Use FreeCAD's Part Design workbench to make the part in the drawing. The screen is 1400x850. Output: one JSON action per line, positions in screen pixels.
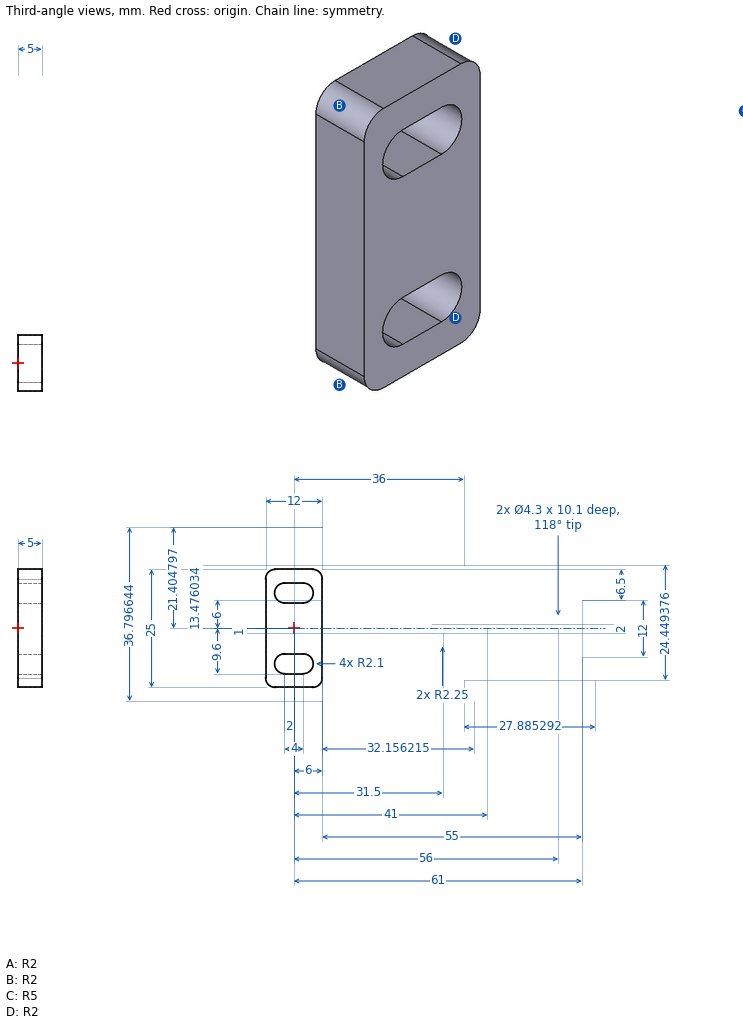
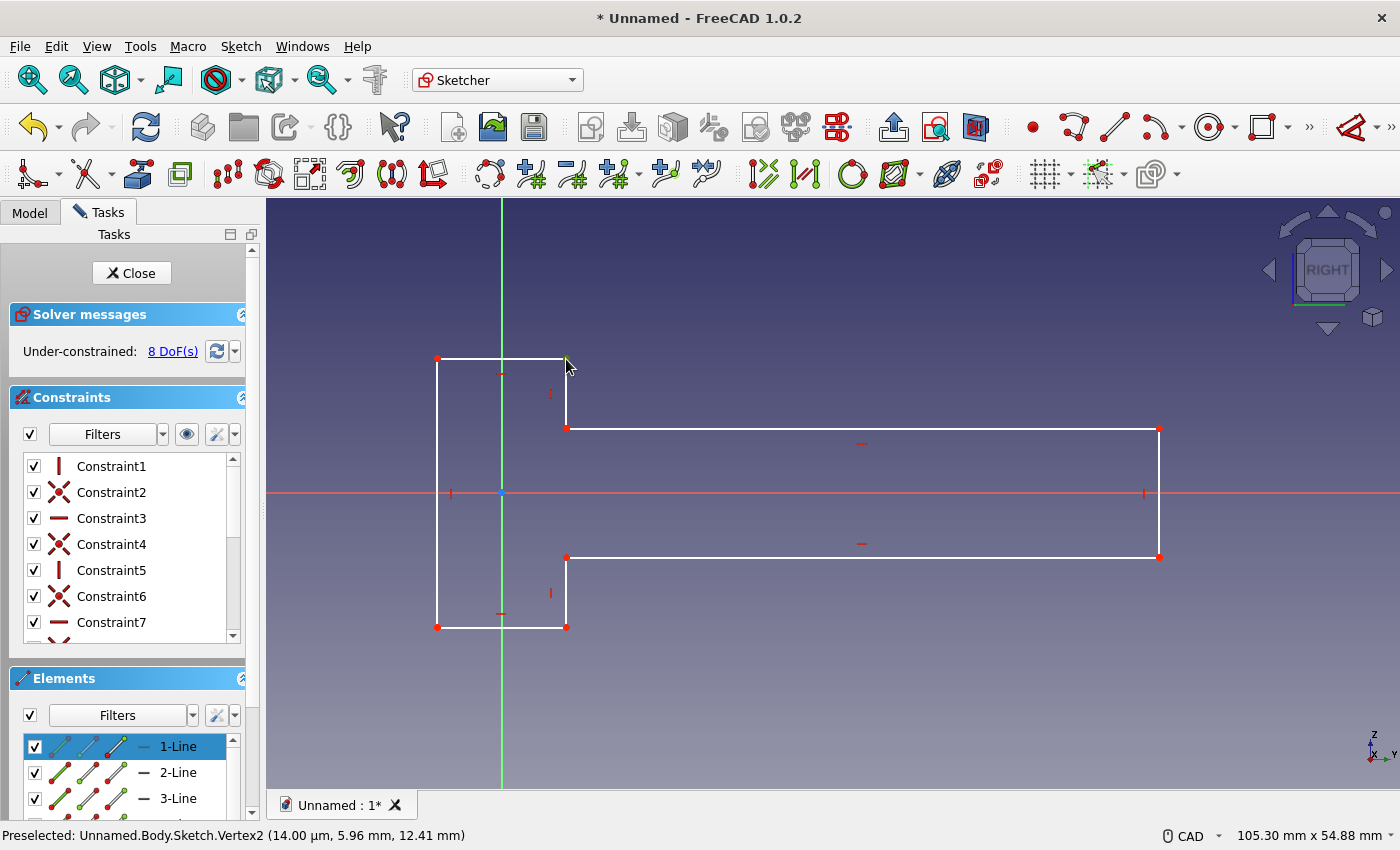
{"action": "left_click", "coordinate": [566, 628]}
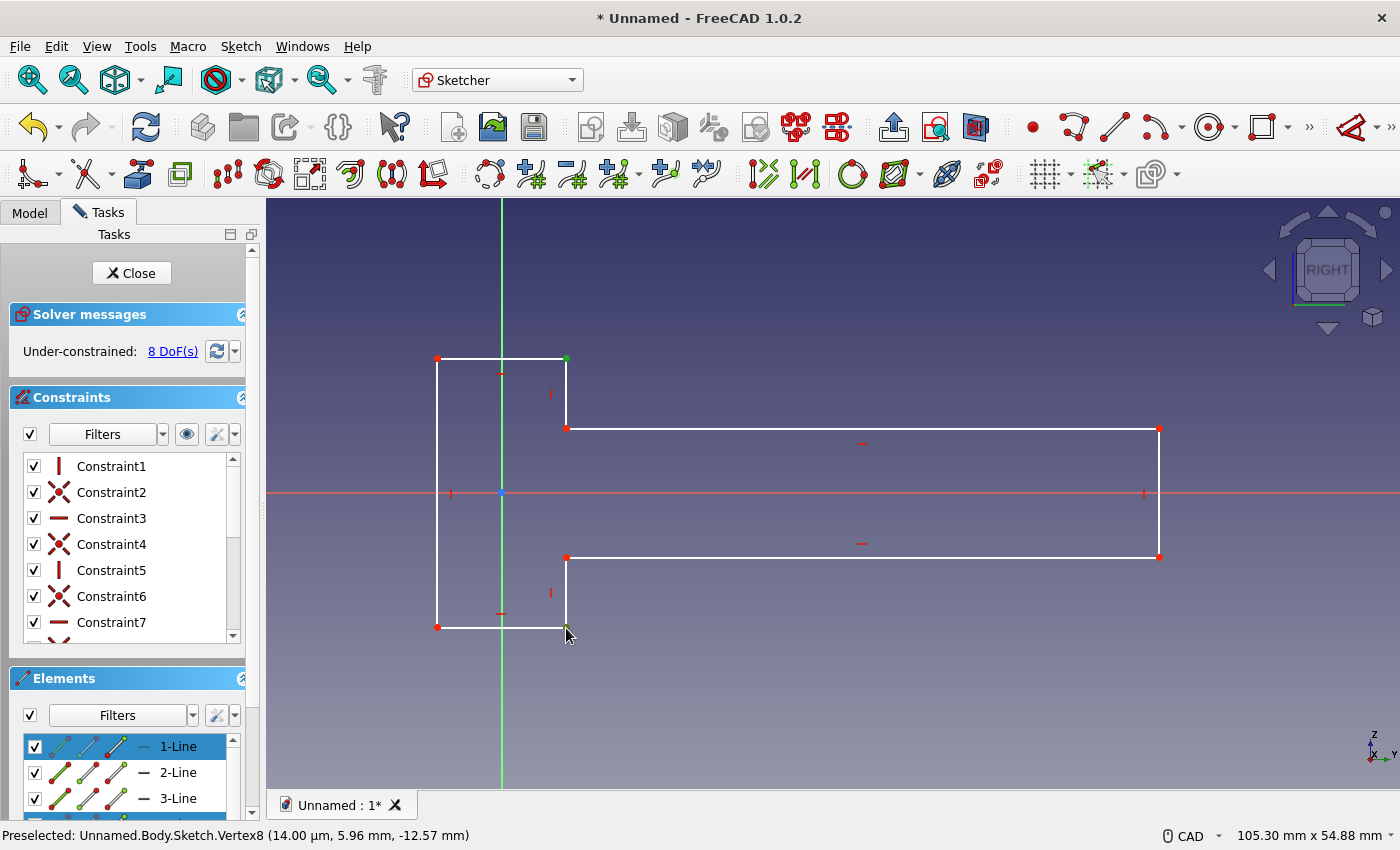
{"action": "left_click", "coordinate": [361, 493]}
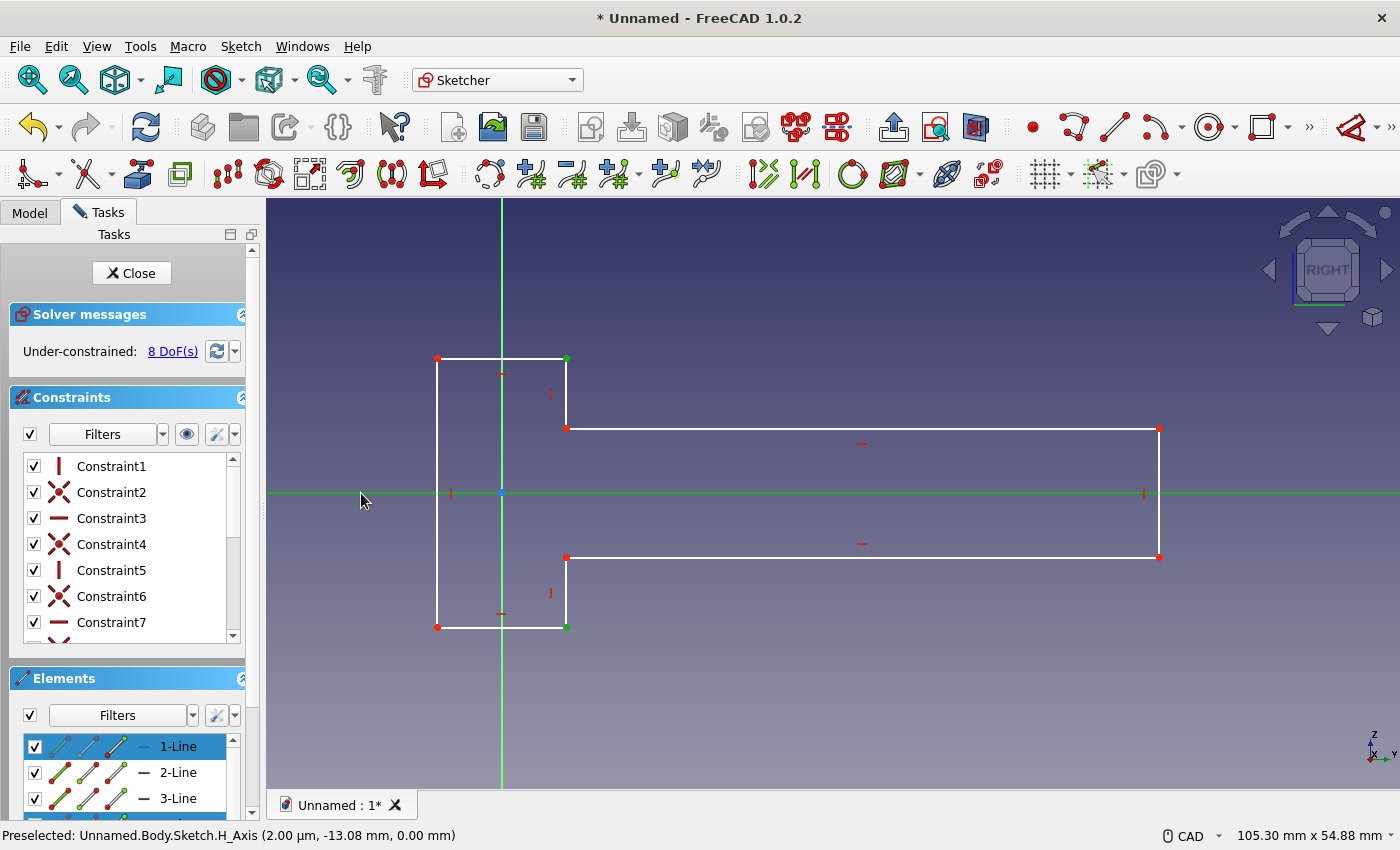
{"action": "key", "text": "s"}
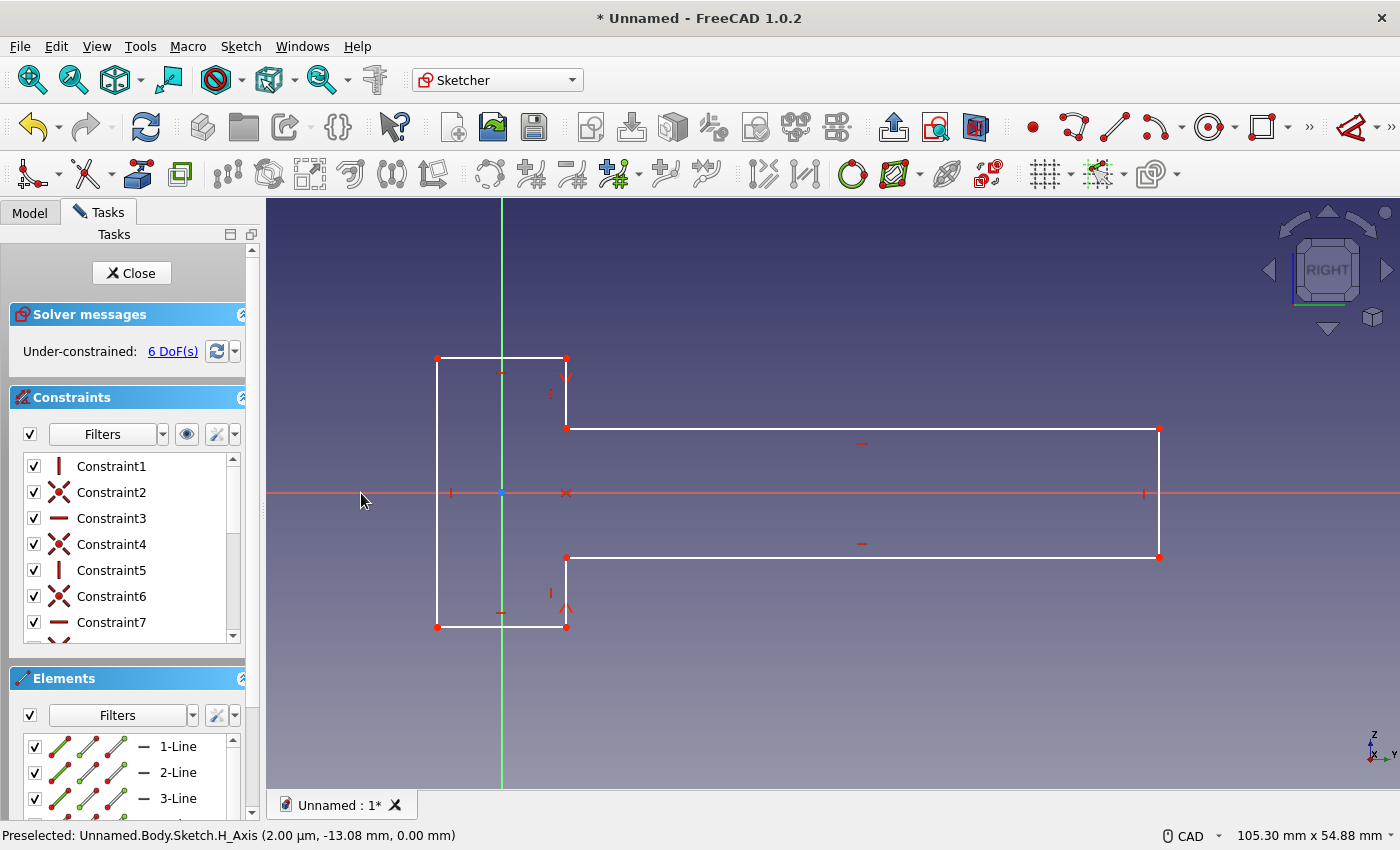
{"action": "left_click", "coordinate": [1350, 128]}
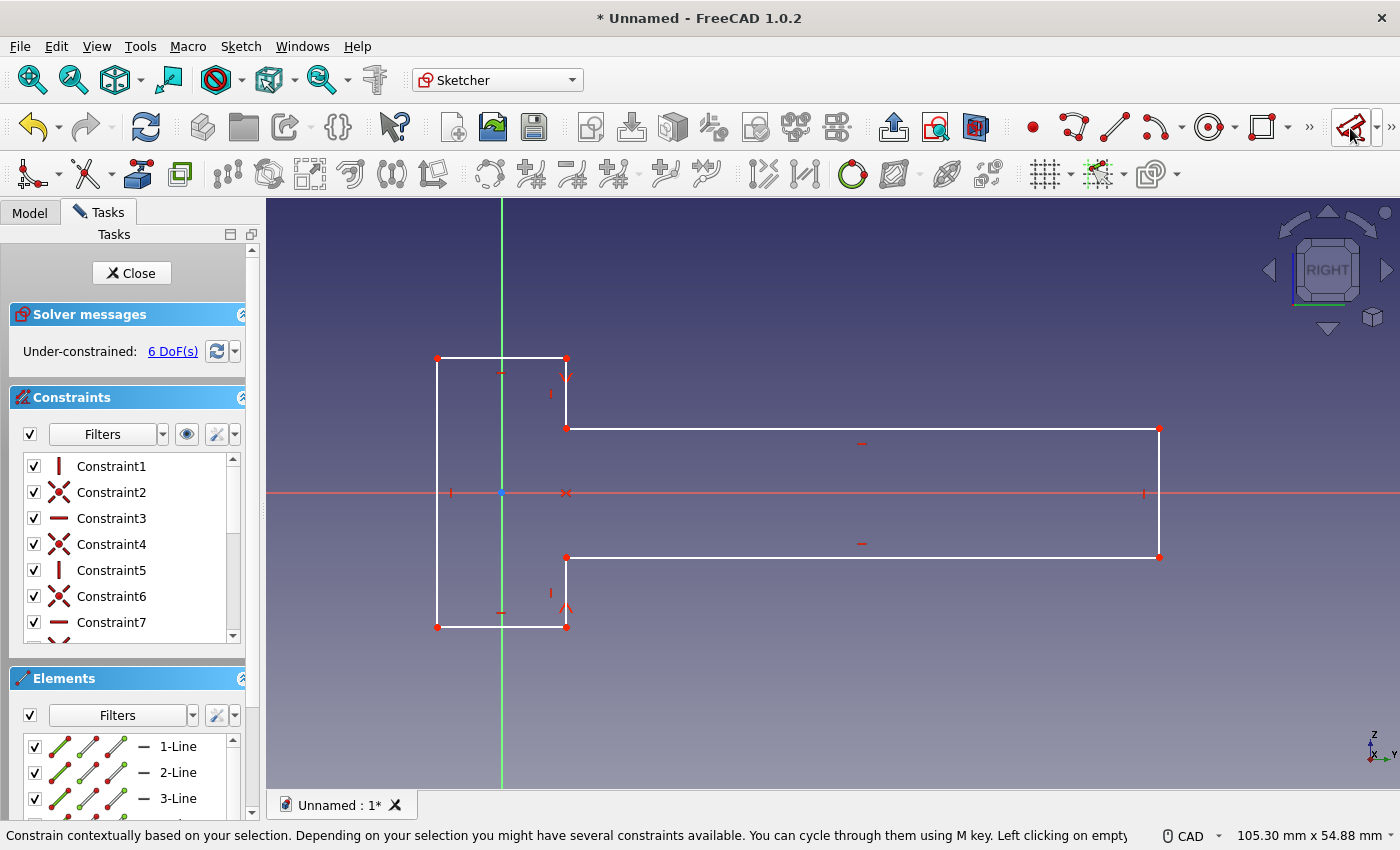
{"action": "left_click", "coordinate": [527, 358]}
{"action": "left_click", "coordinate": [472, 324]}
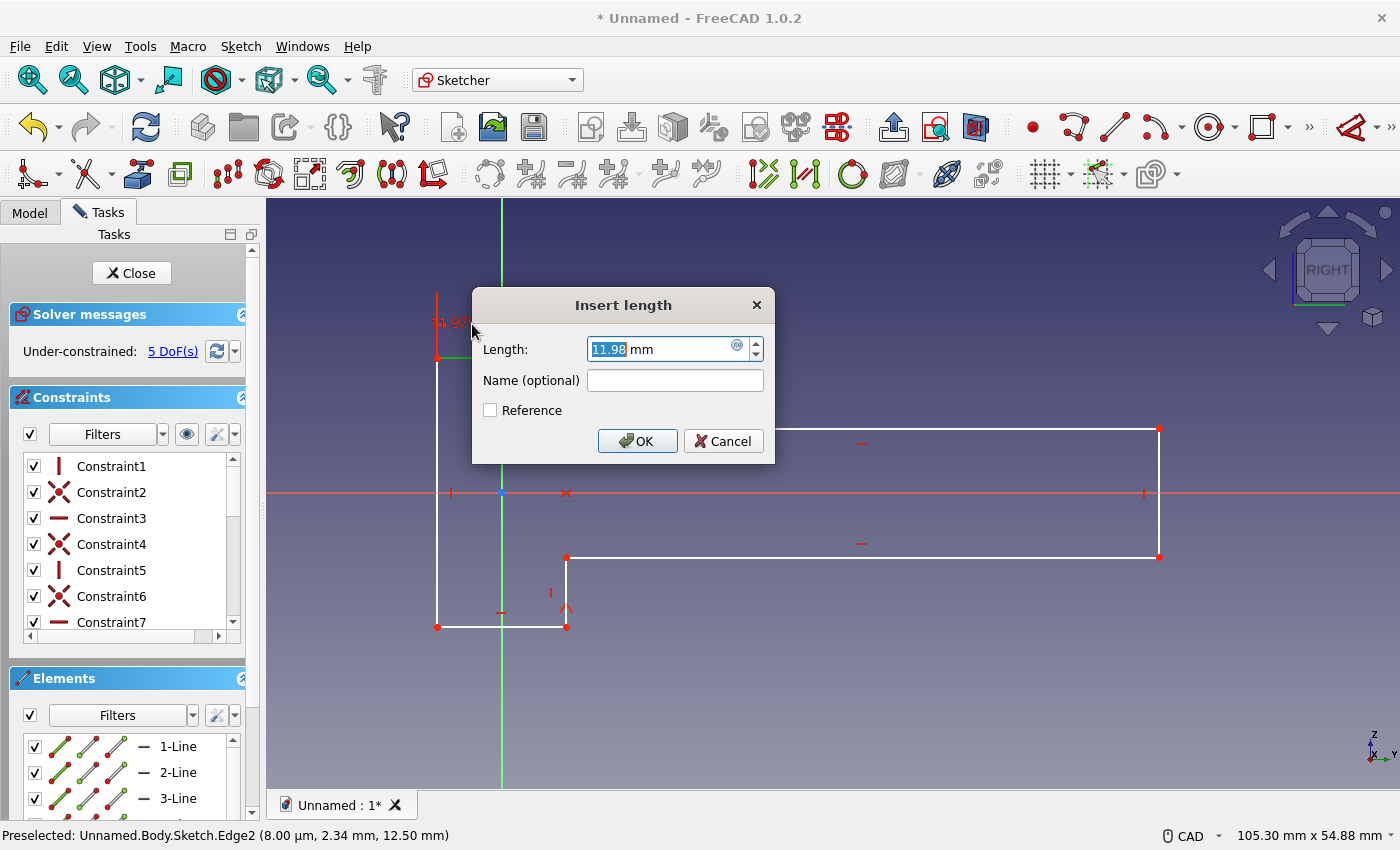
{"action": "type", "text": "12"}
{"action": "key", "text": "Return"}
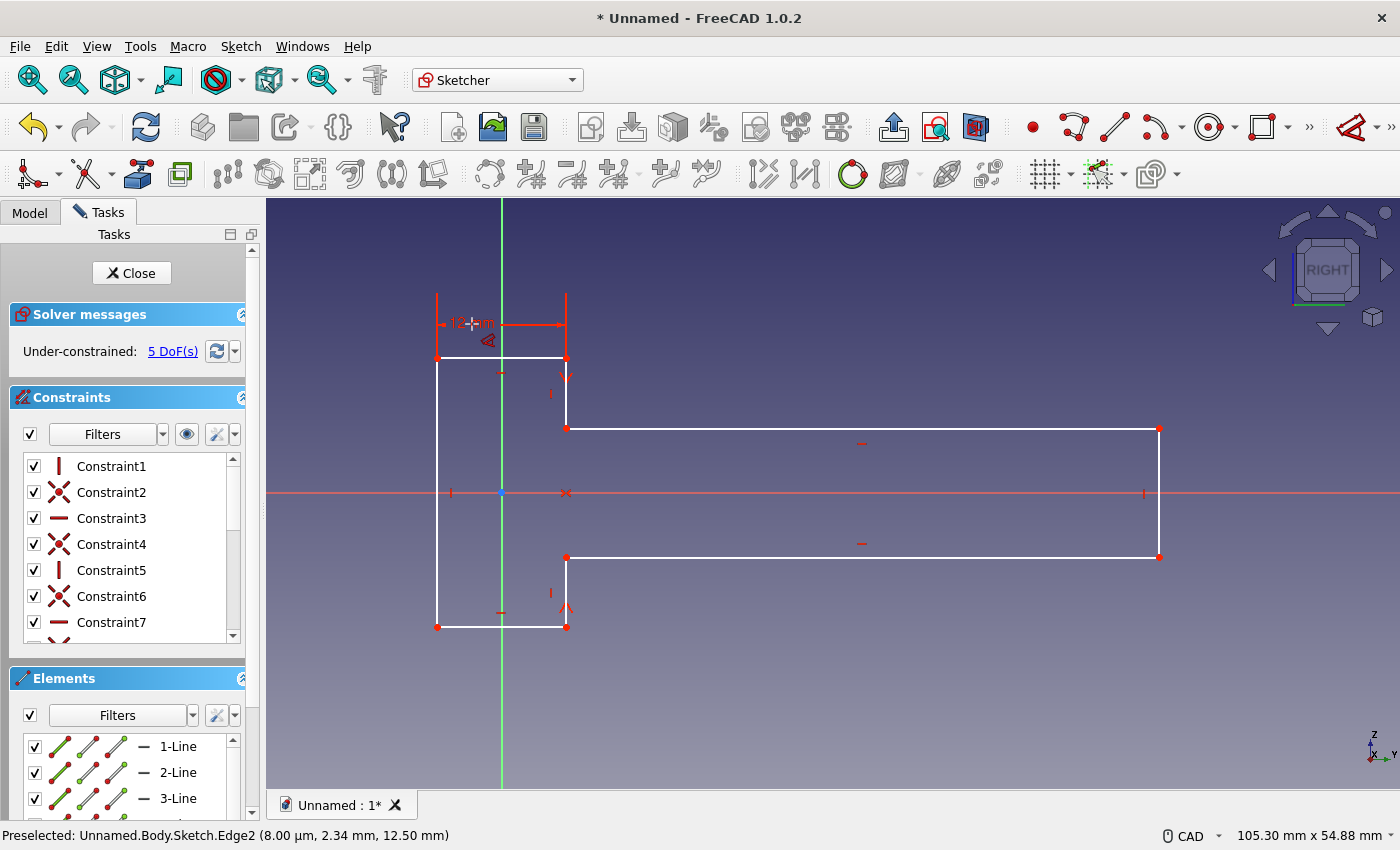
{"action": "left_click", "coordinate": [437, 439]}
{"action": "left_click", "coordinate": [403, 431]}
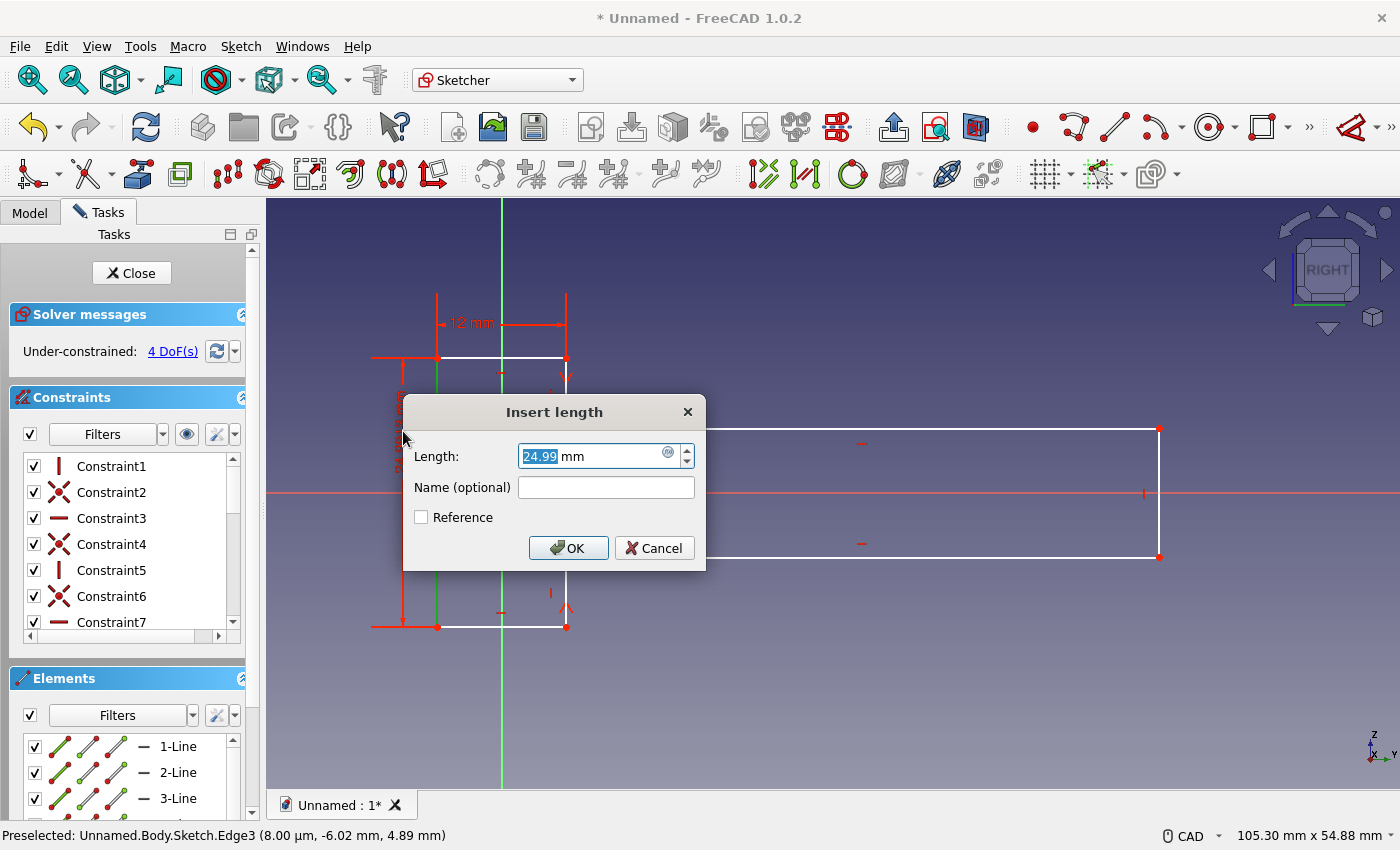
{"action": "type", "text": "25"}
{"action": "key", "text": "Return"}